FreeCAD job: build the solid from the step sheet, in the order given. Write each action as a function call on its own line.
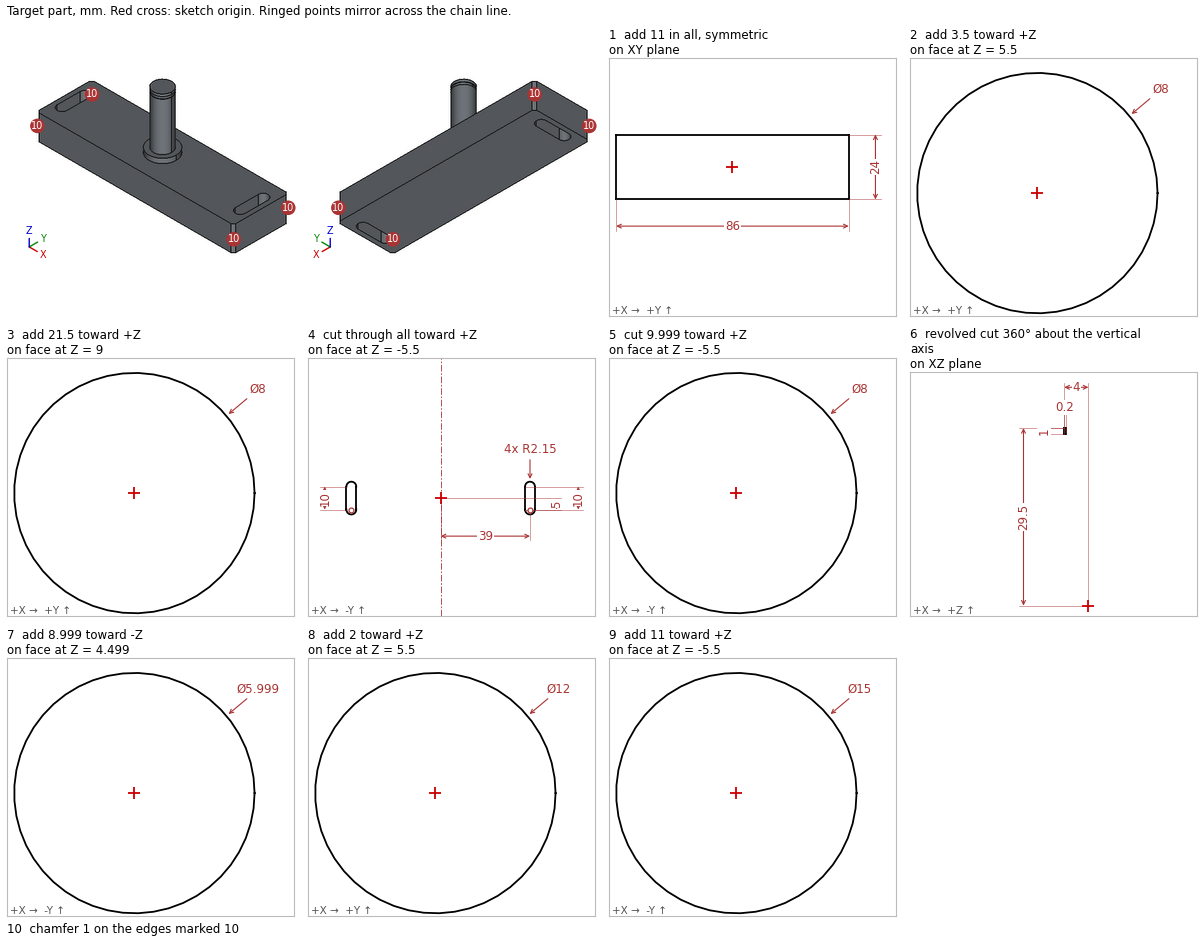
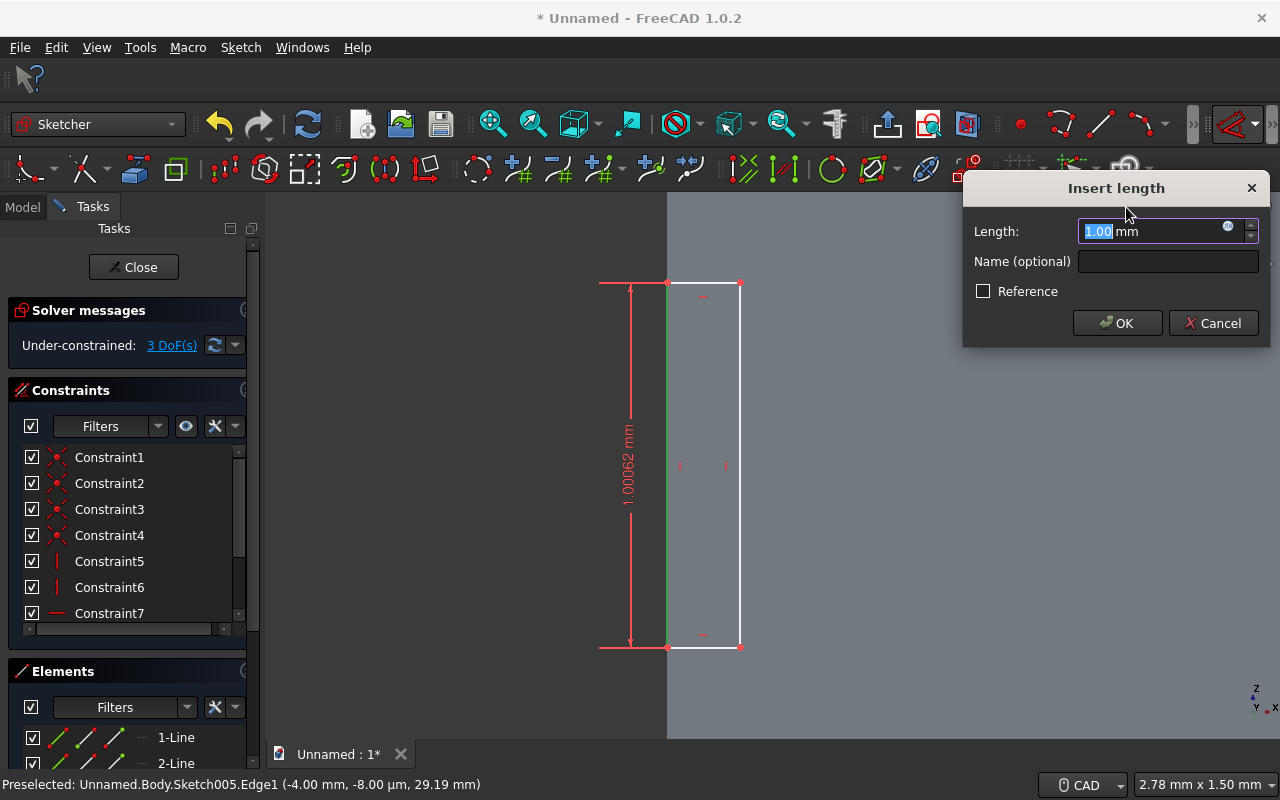
text(1)
key(Return)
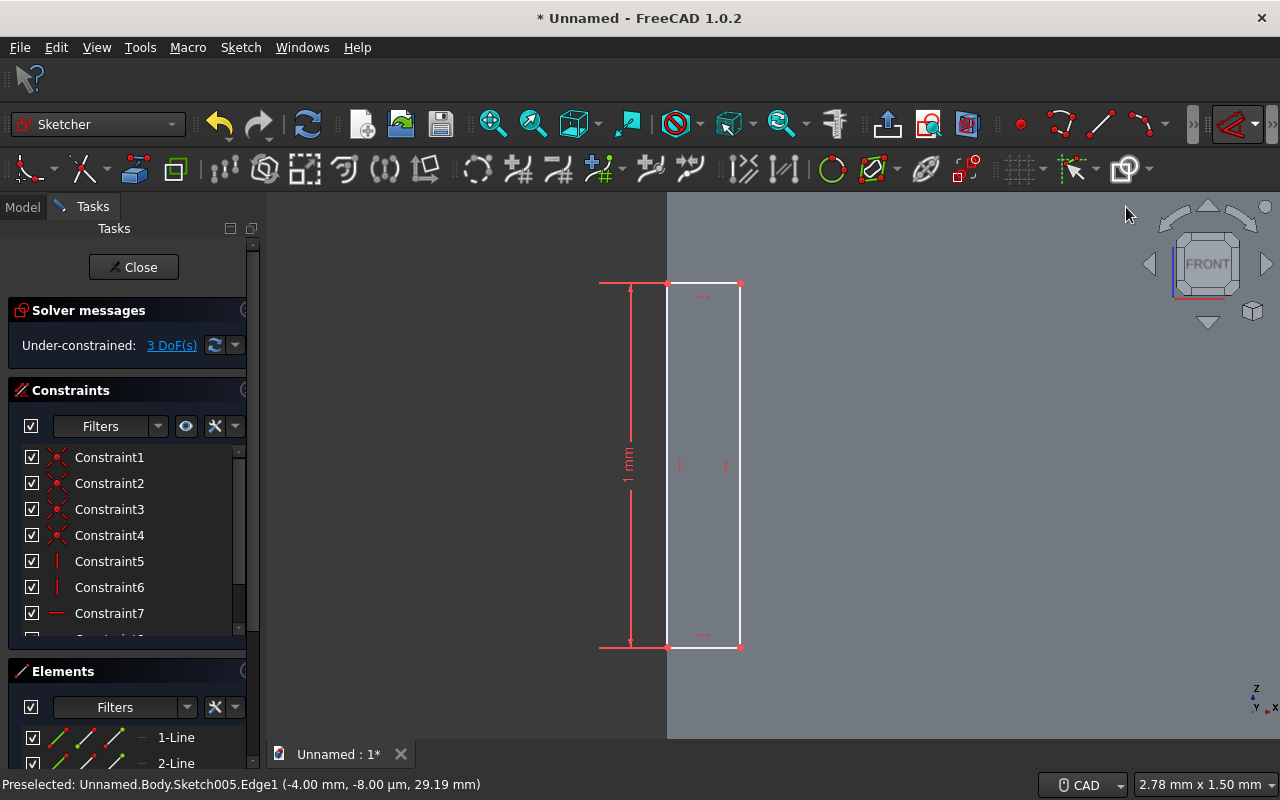
click(667, 283)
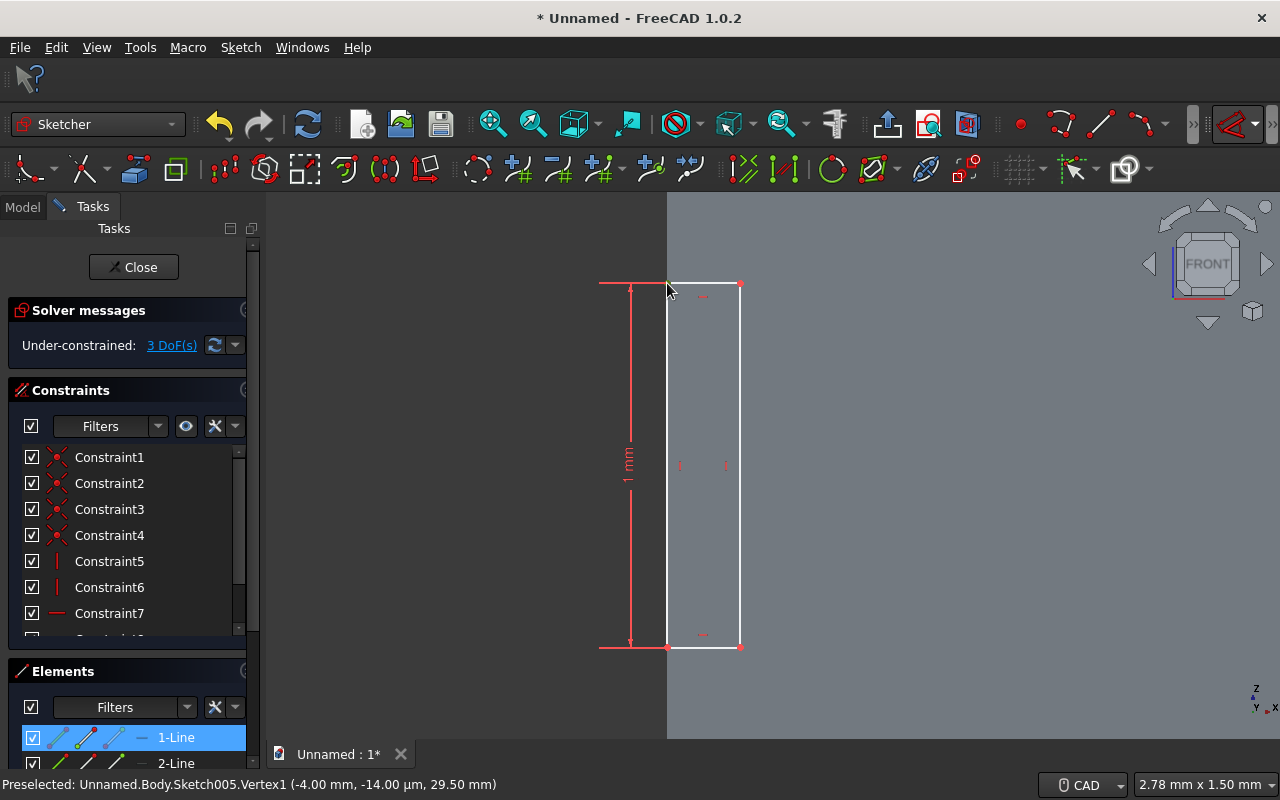
key(l)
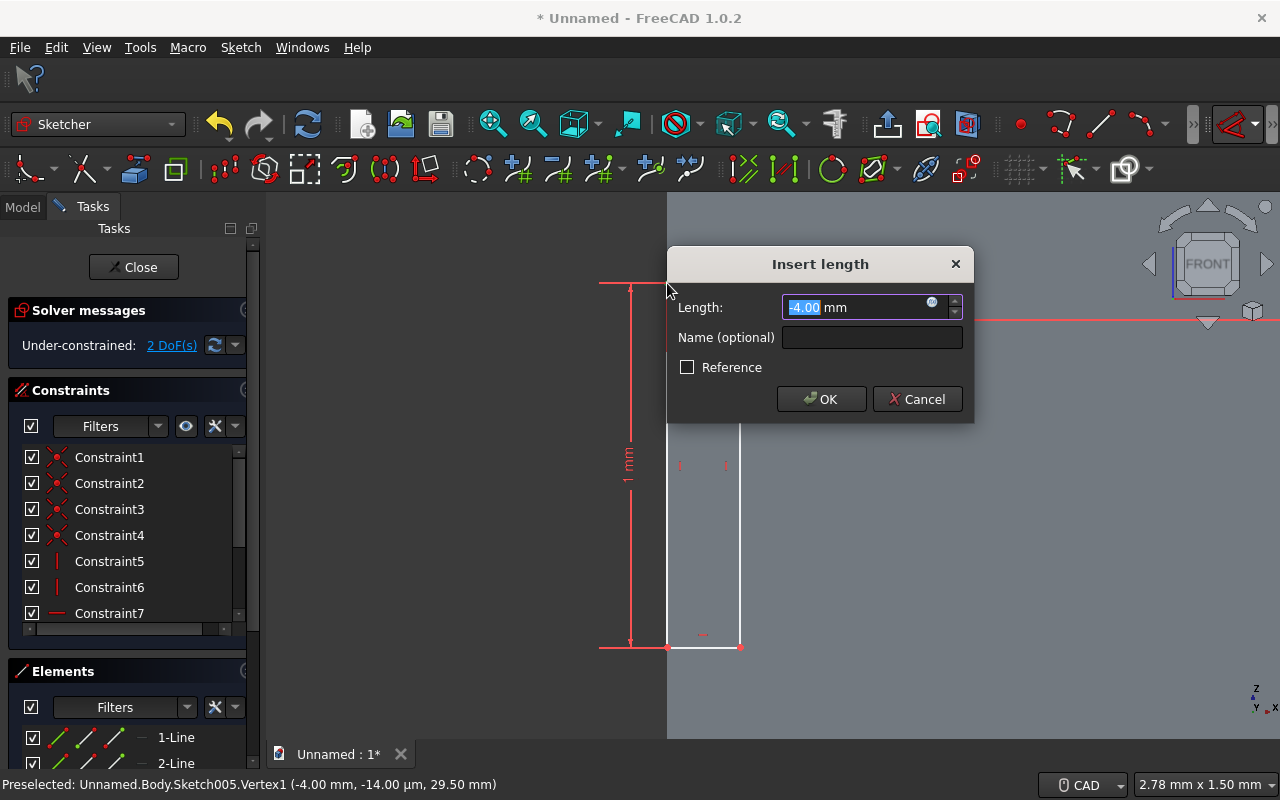
text(-4)
key(Return)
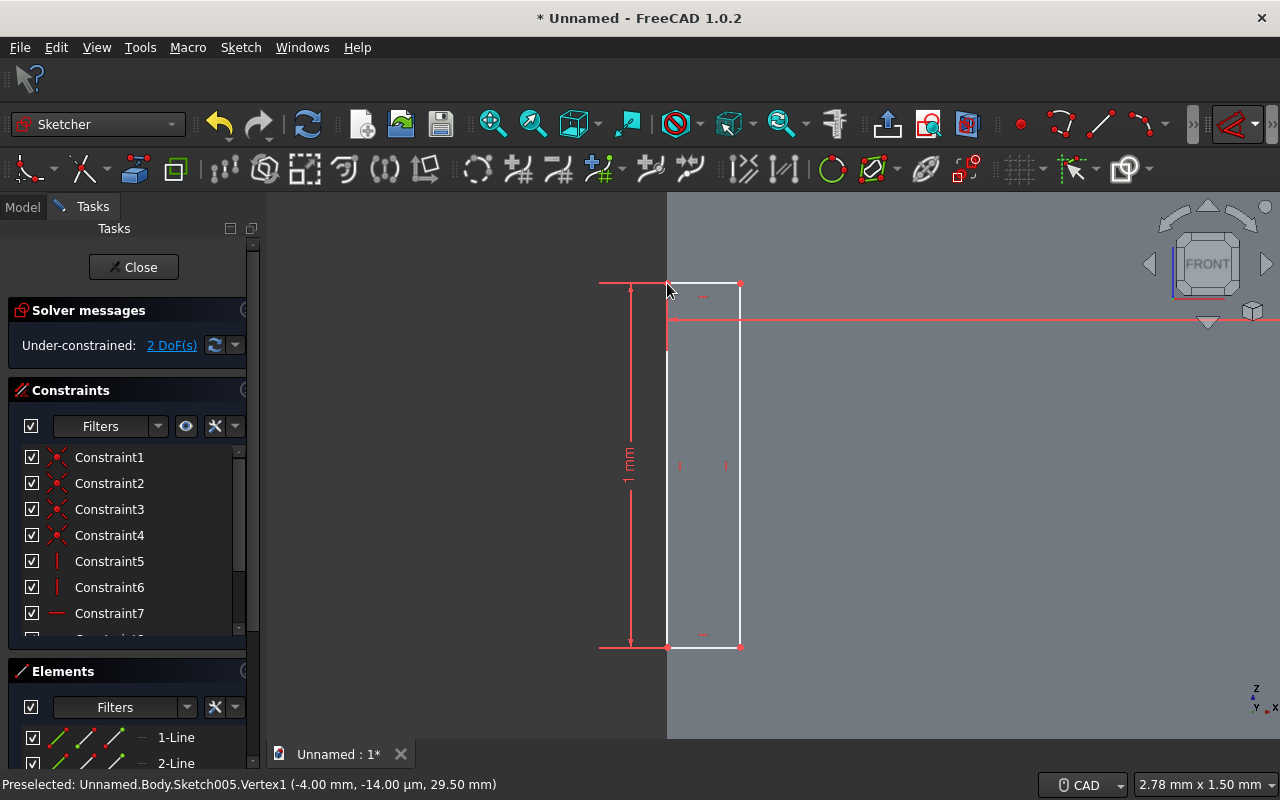
click(689, 648)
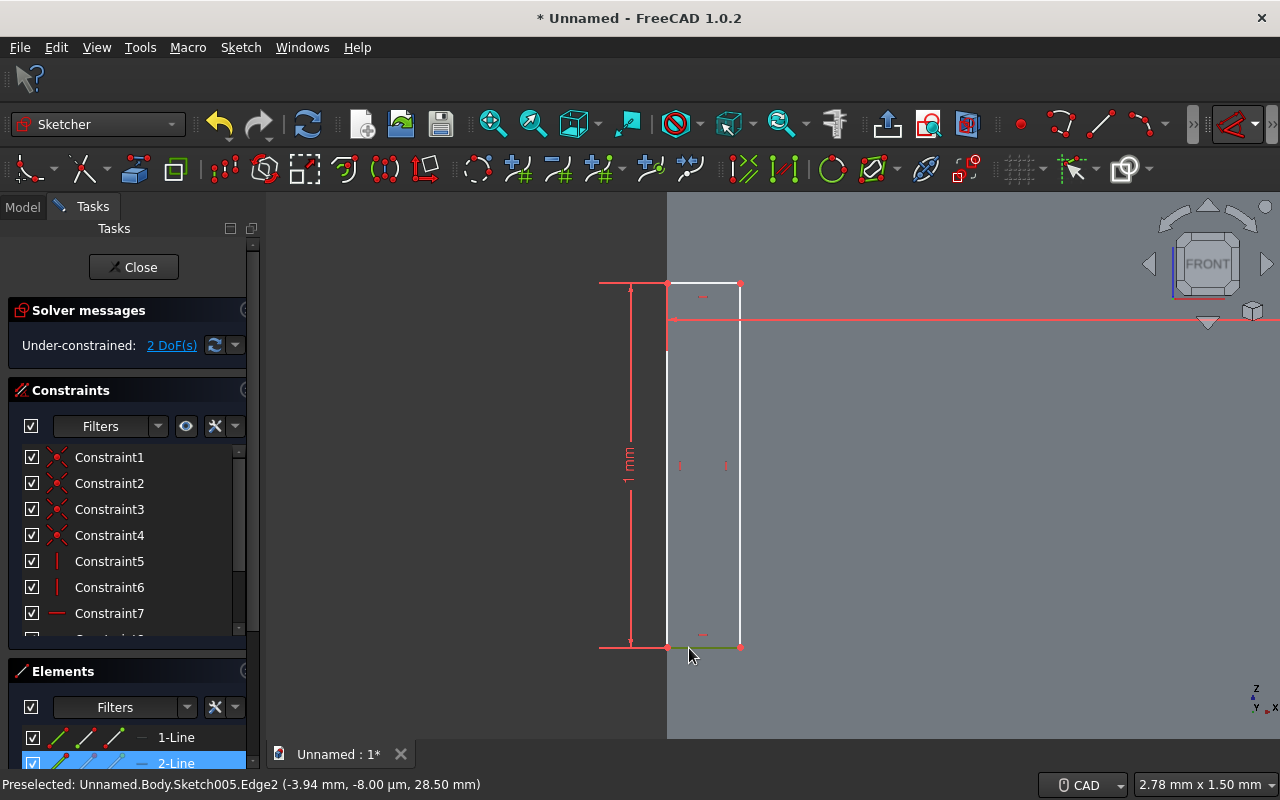
click(1258, 124)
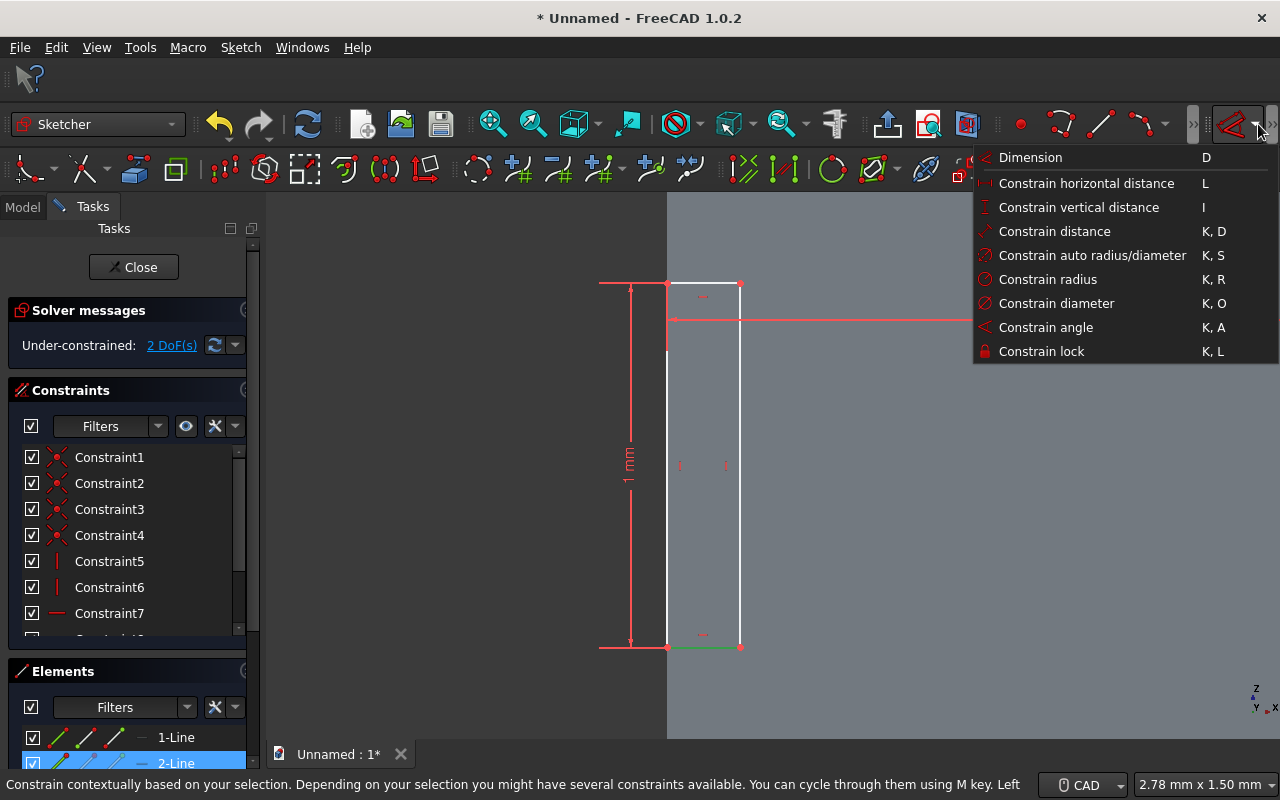
click(1126, 183)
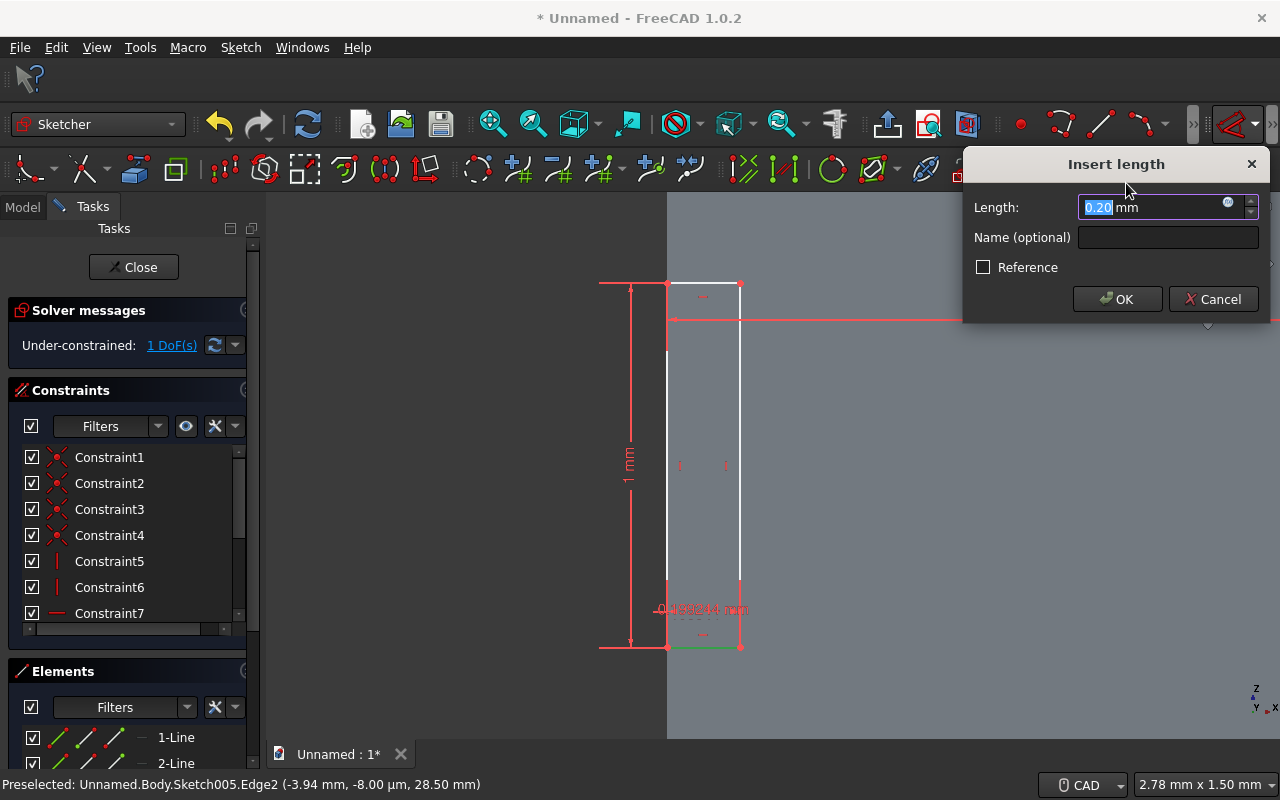
text(0.2)
key(Return)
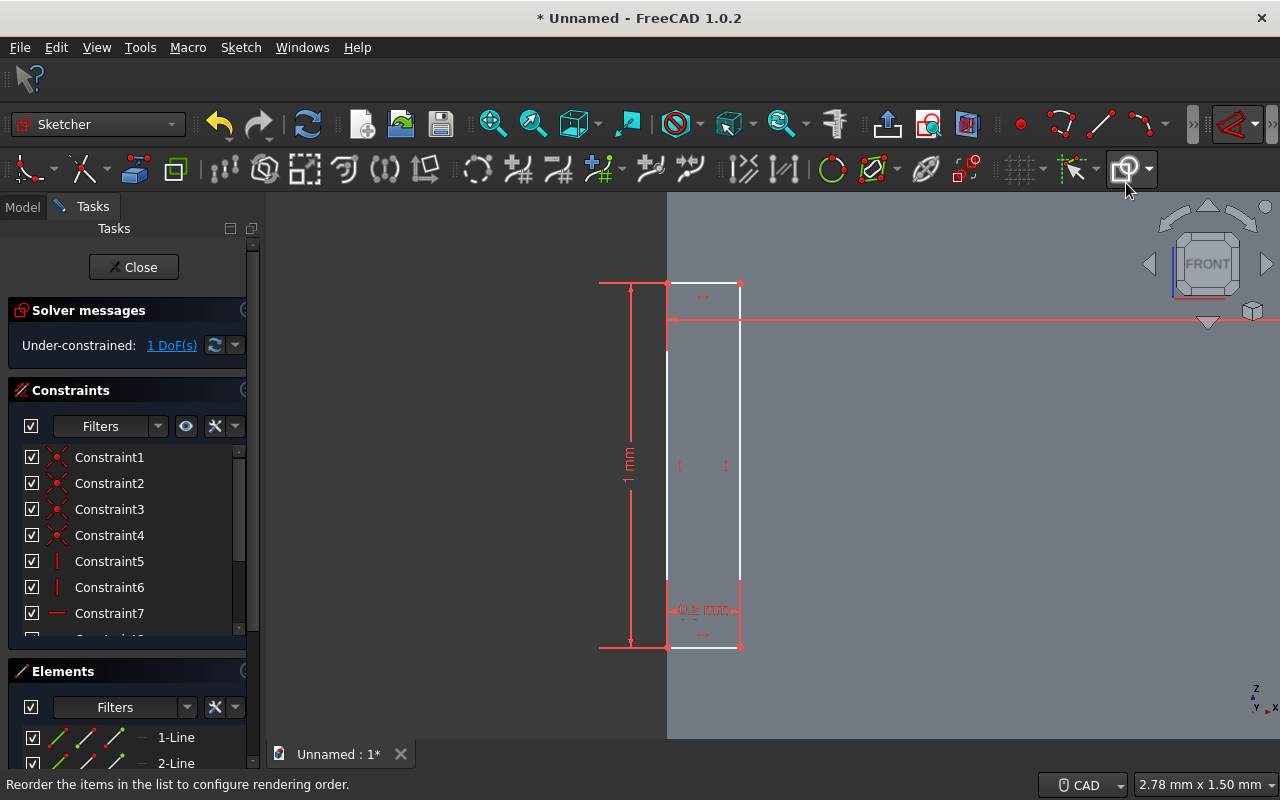
click(667, 283)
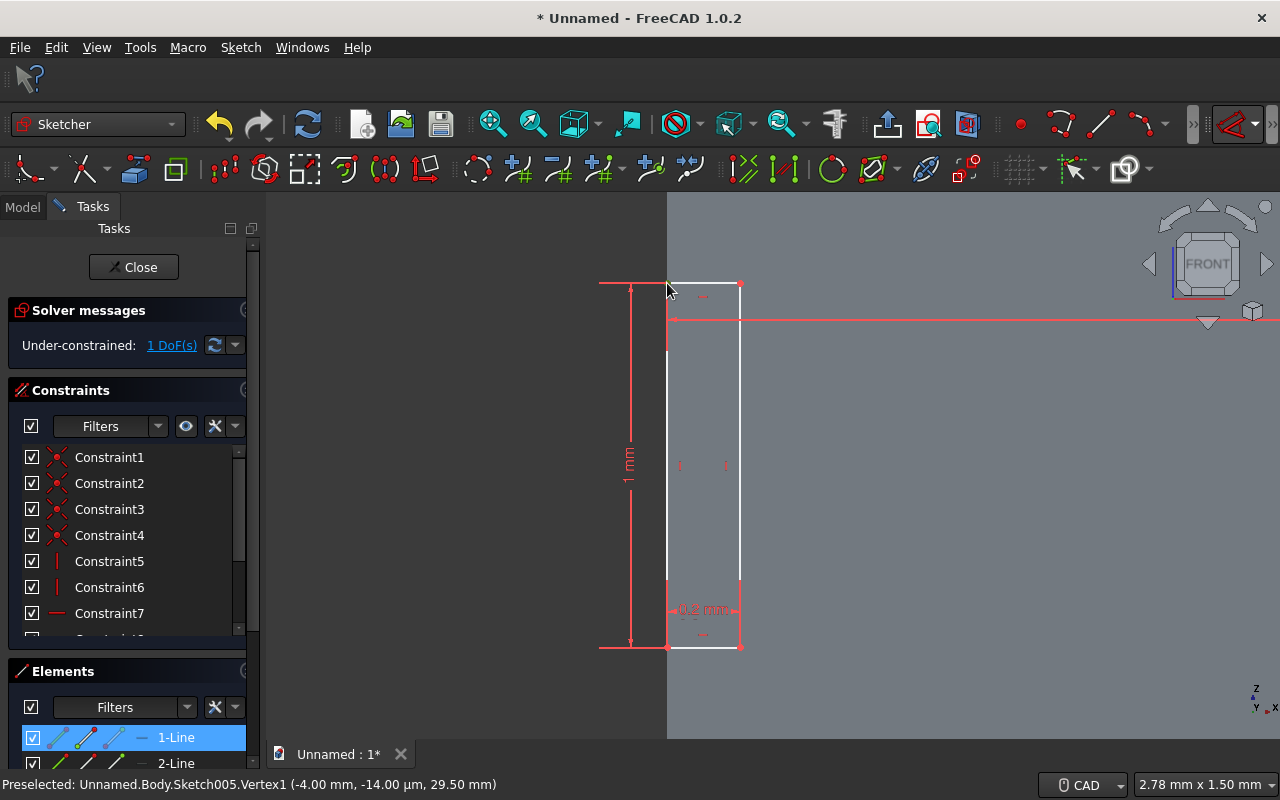
key(i)